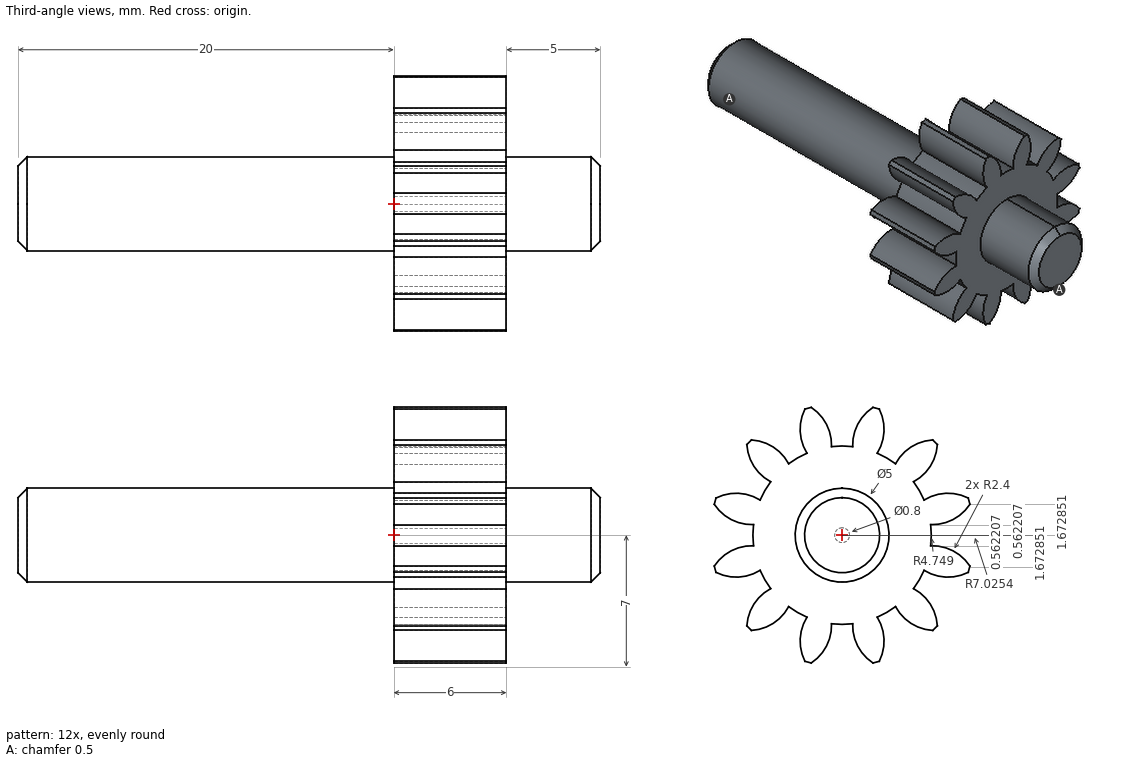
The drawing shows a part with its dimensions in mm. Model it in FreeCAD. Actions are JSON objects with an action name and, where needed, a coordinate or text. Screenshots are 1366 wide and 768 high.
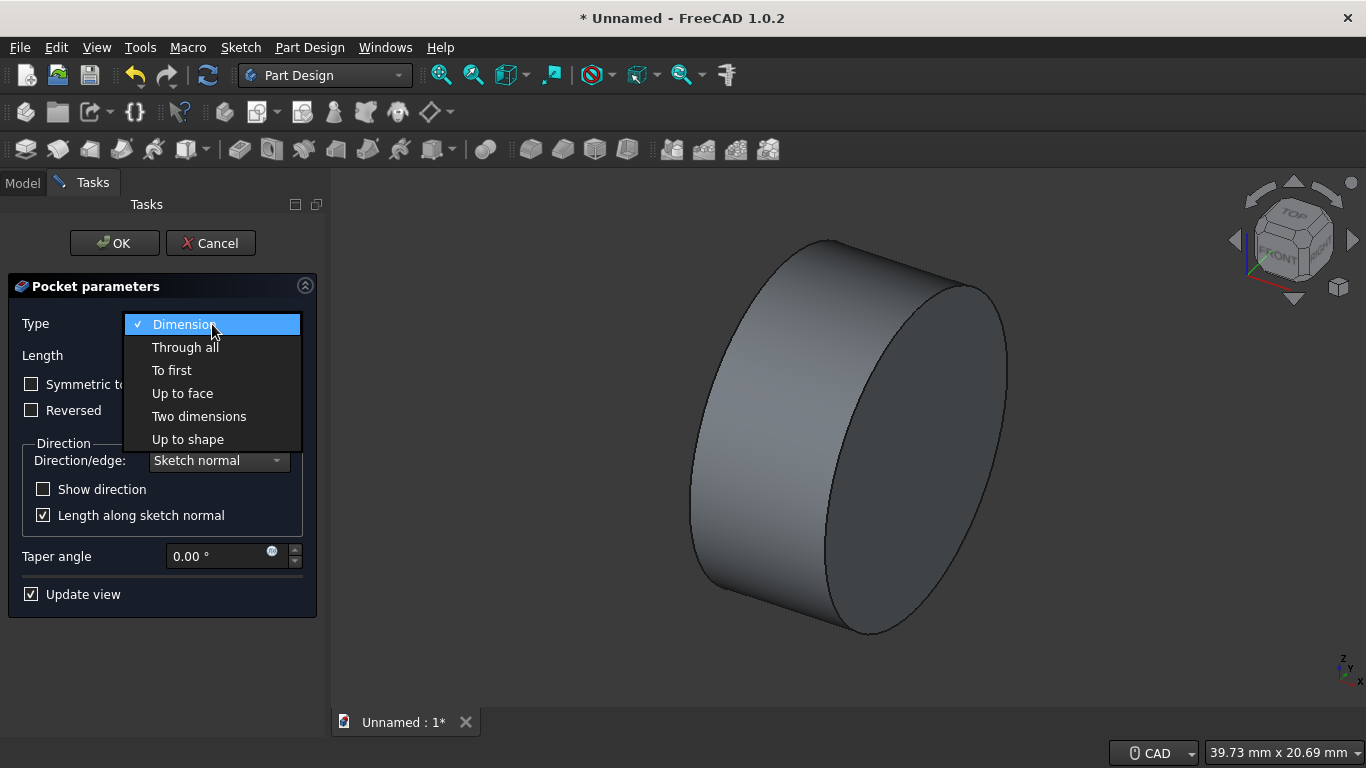
{"action": "left_click", "coordinate": [212, 348]}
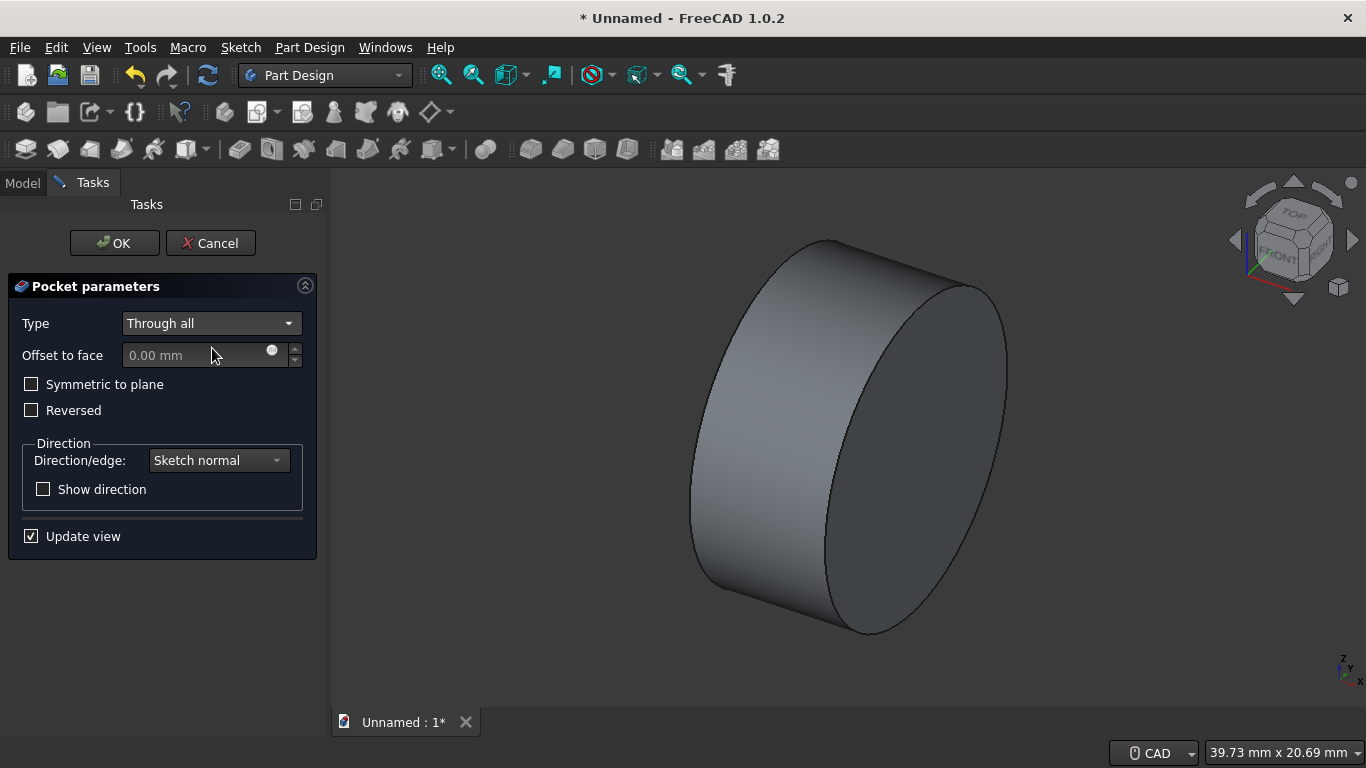
{"action": "left_click", "coordinate": [30, 410]}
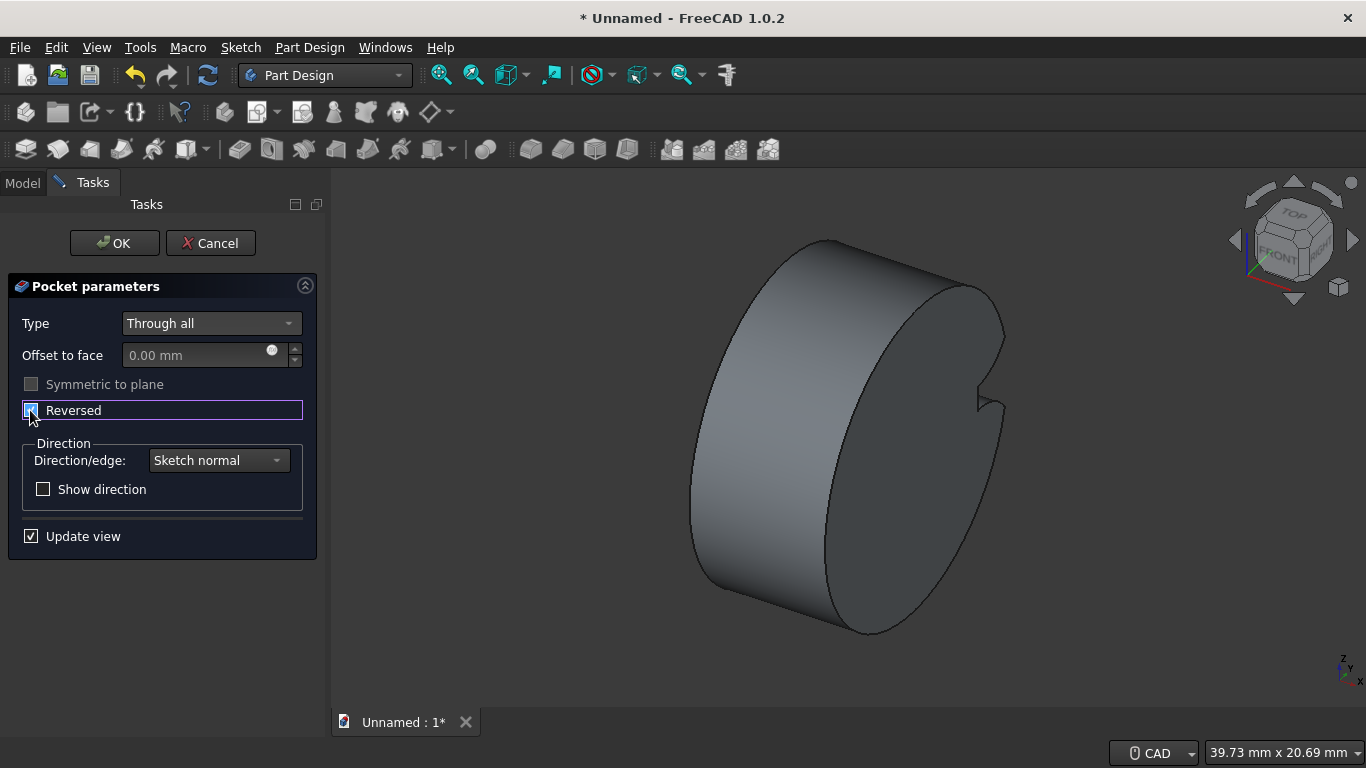
{"action": "left_click", "coordinate": [115, 243]}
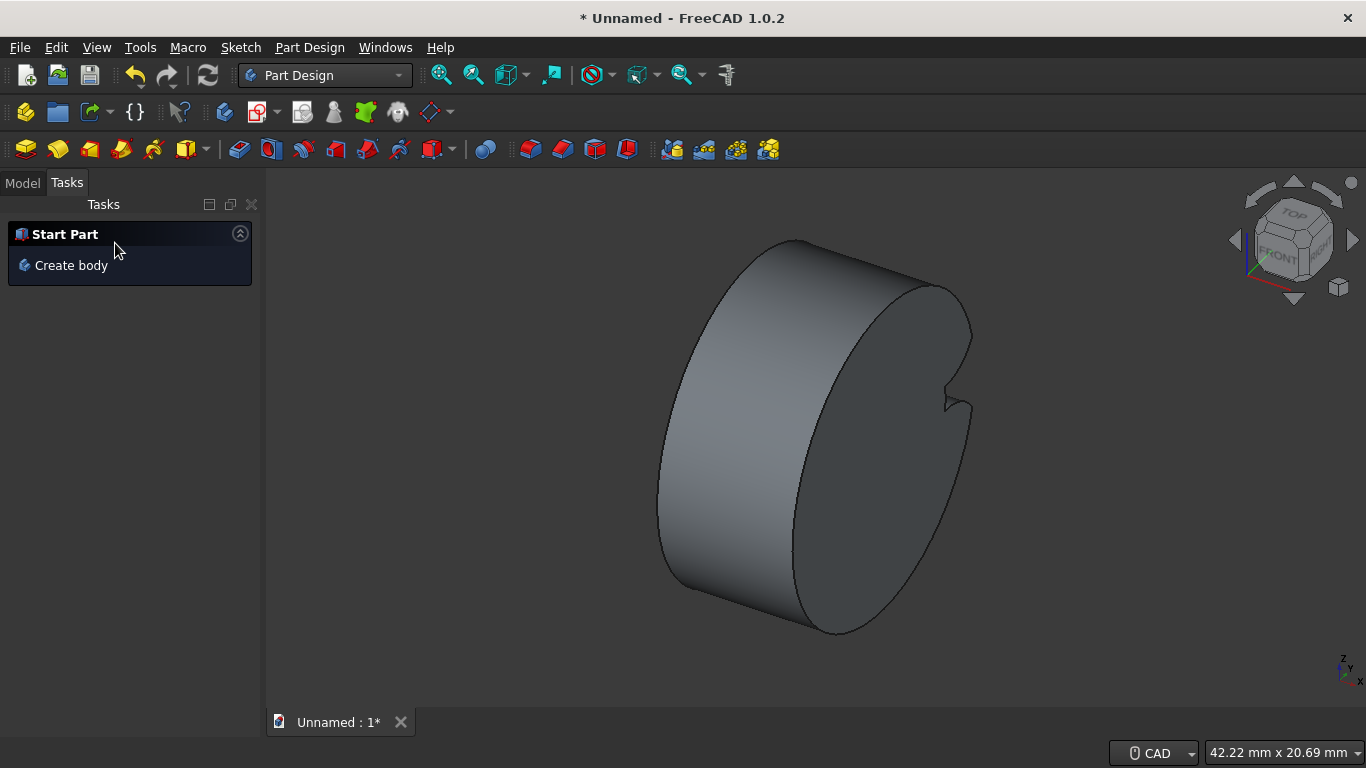
{"action": "left_click", "coordinate": [23, 182]}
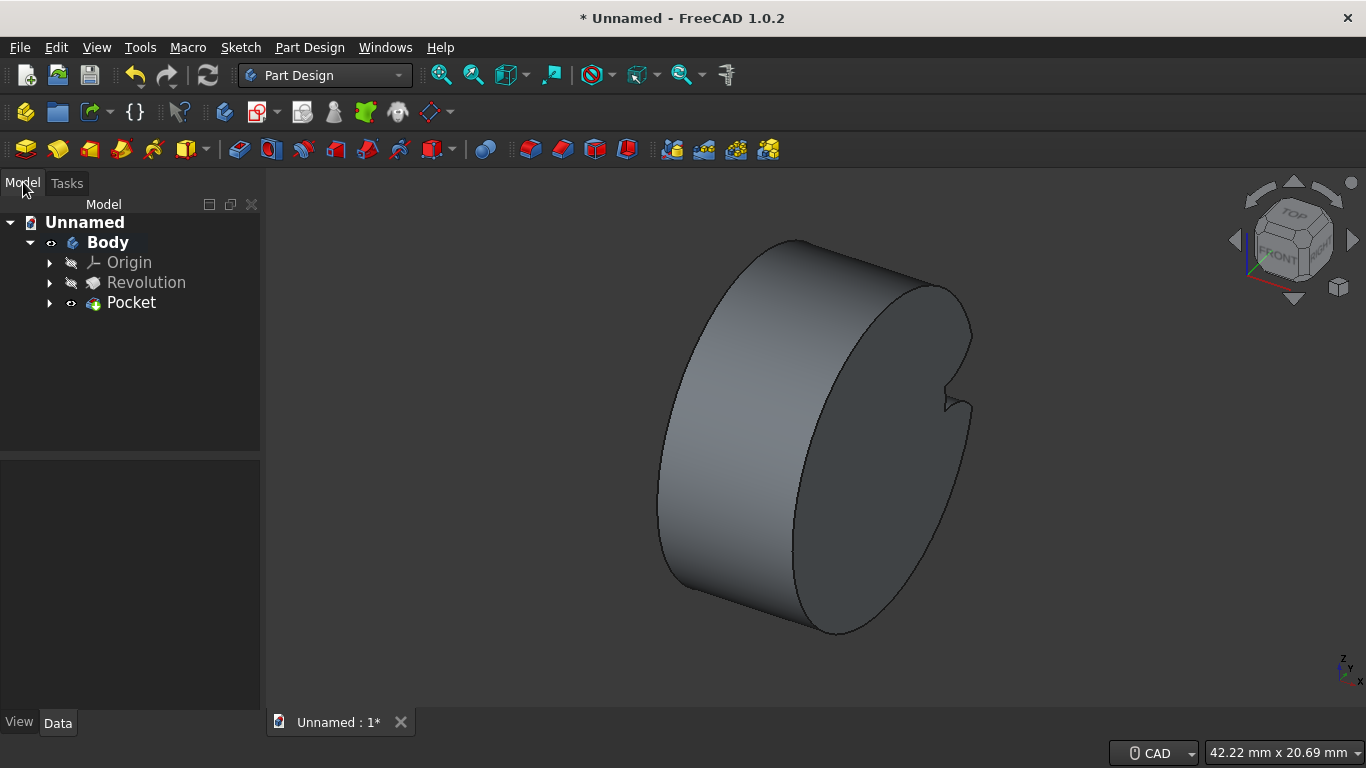
{"action": "left_click", "coordinate": [116, 303]}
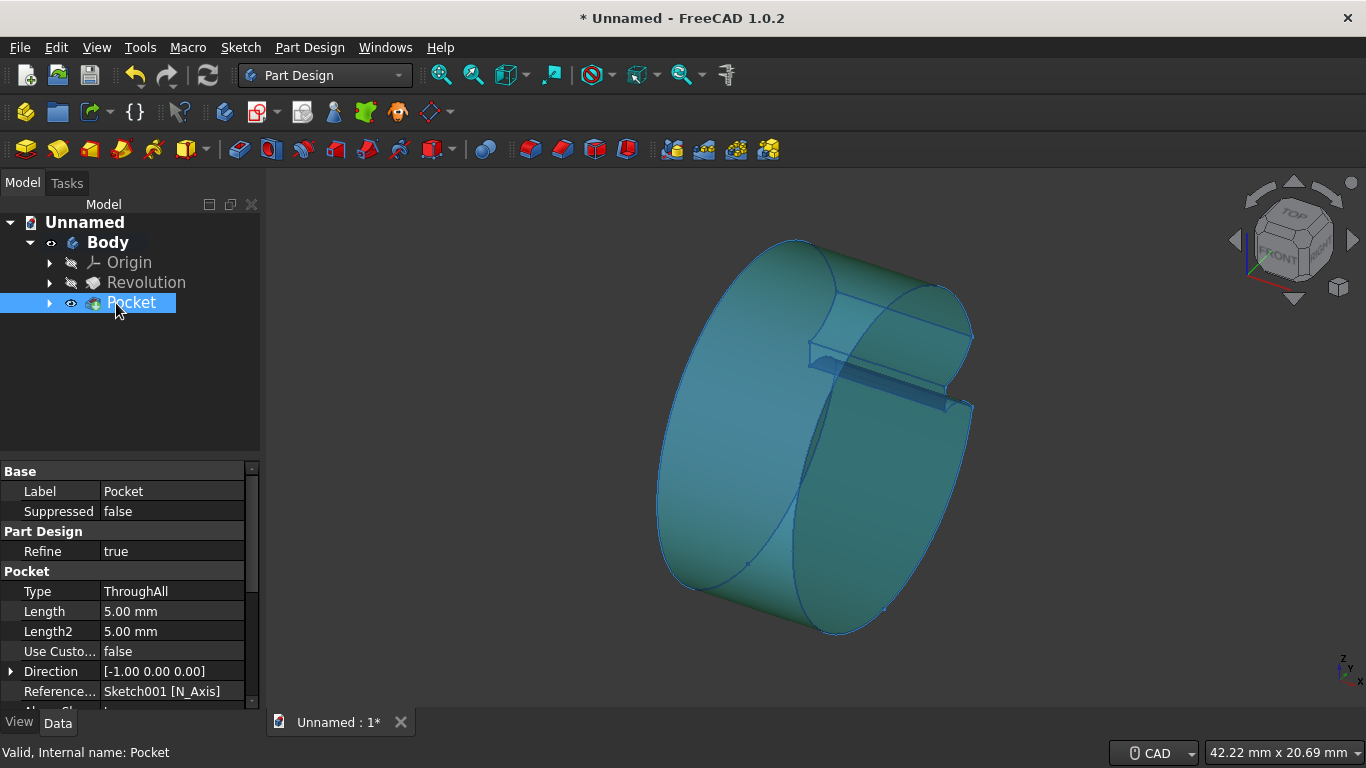
{"action": "left_click", "coordinate": [736, 150]}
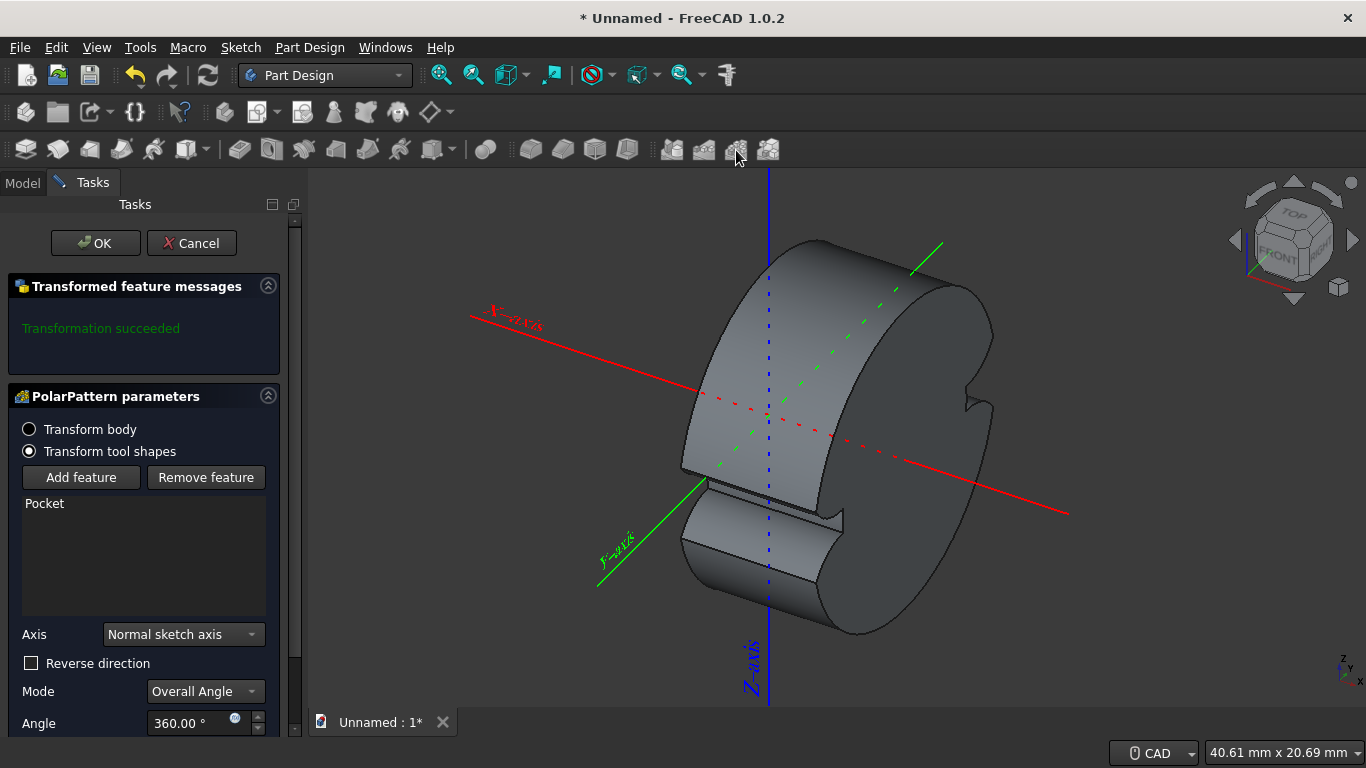
{"action": "left_click", "coordinate": [184, 634]}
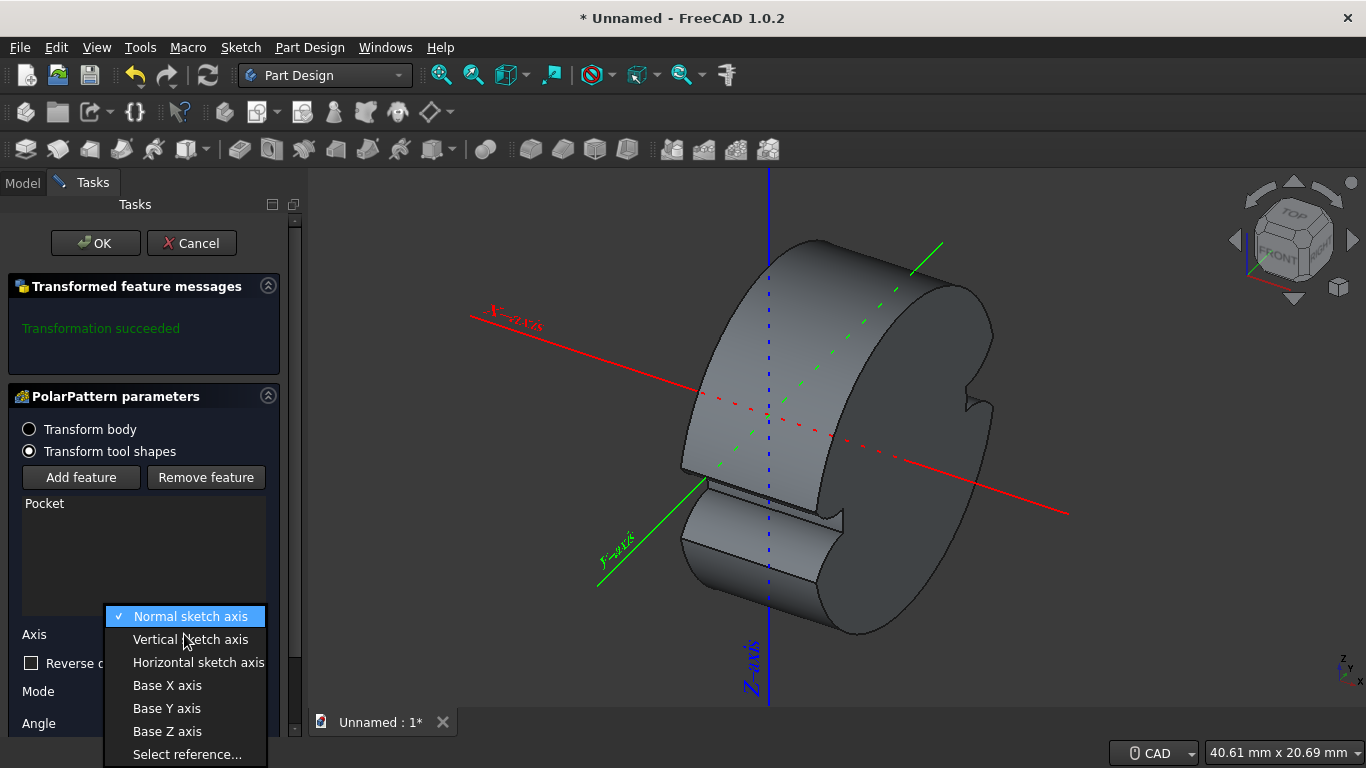
{"action": "left_click", "coordinate": [184, 686]}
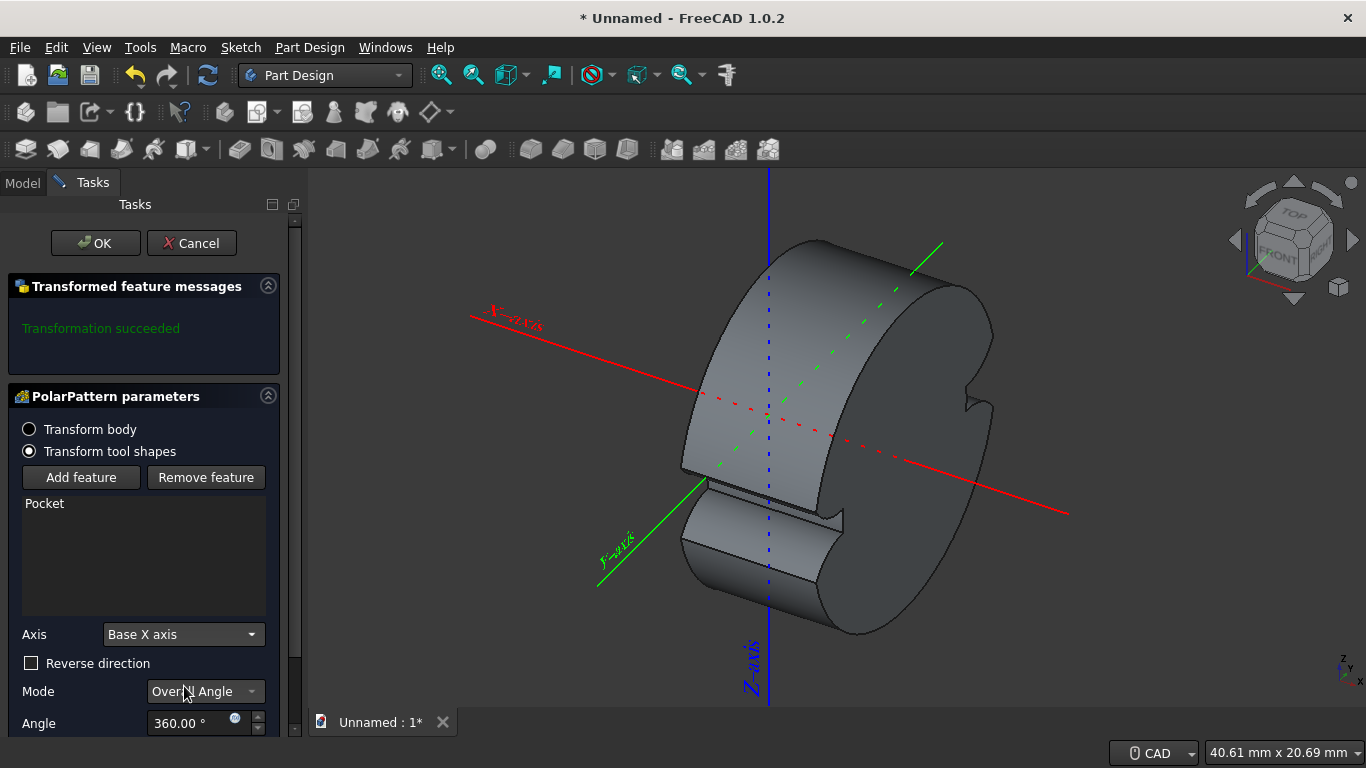
{"action": "scroll", "coordinate": [295, 475], "scroll_direction": "down", "scroll_amount": 2}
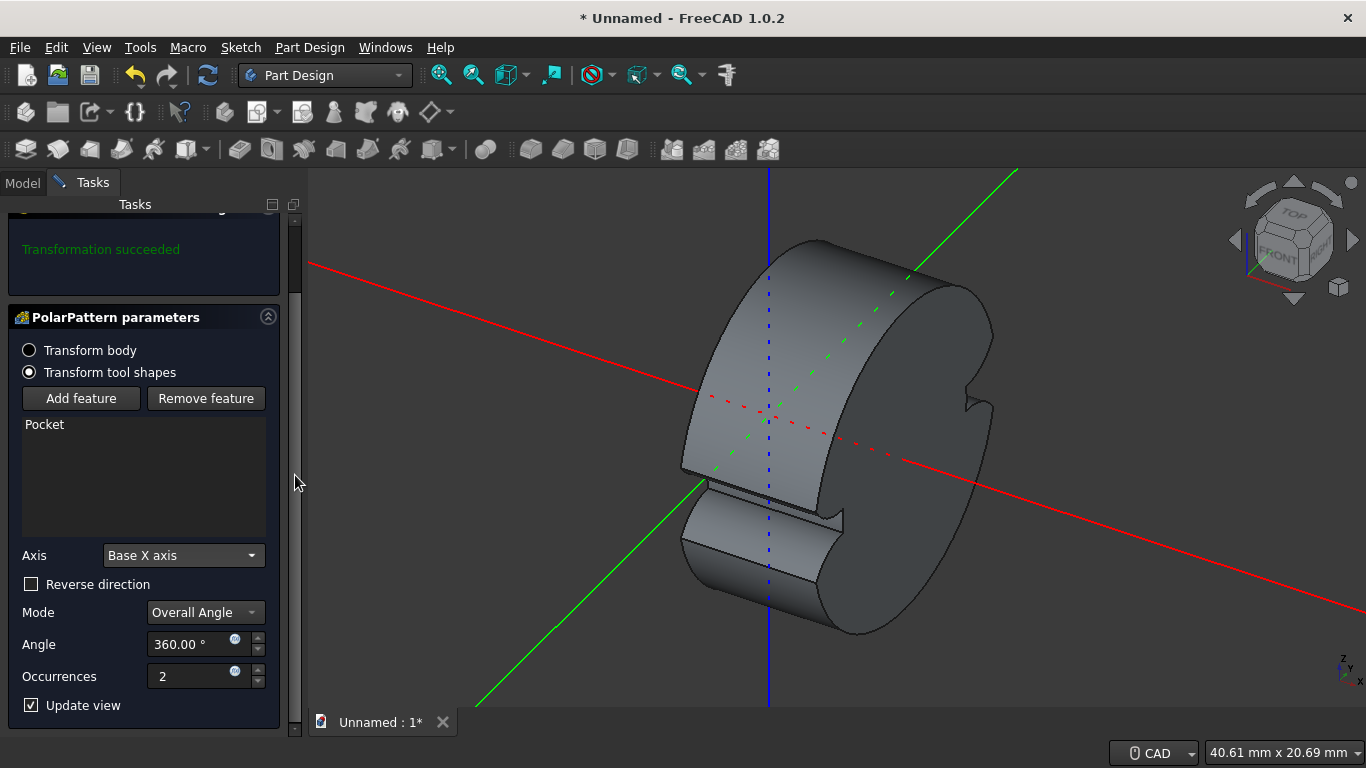
{"action": "triple_click", "coordinate": [198, 676]}